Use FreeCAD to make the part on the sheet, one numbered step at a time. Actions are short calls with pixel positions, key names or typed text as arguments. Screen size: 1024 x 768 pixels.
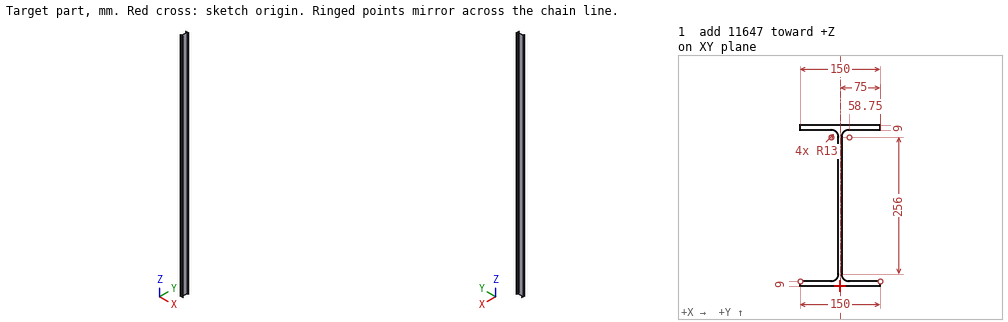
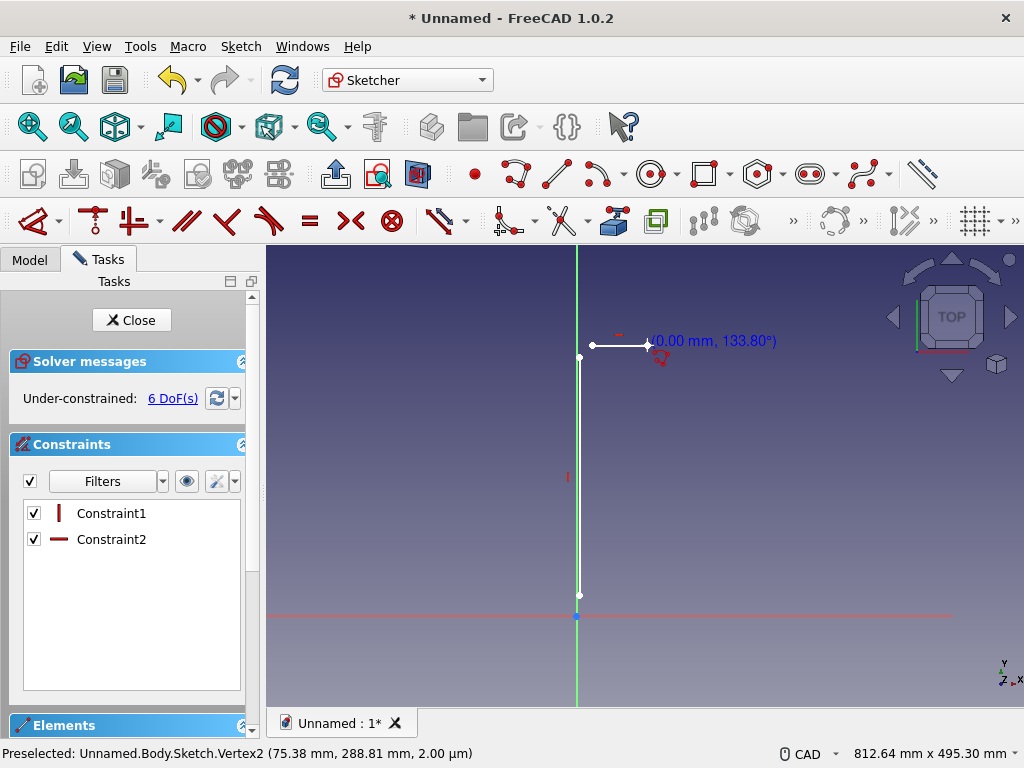
scroll(647, 337, up, 4)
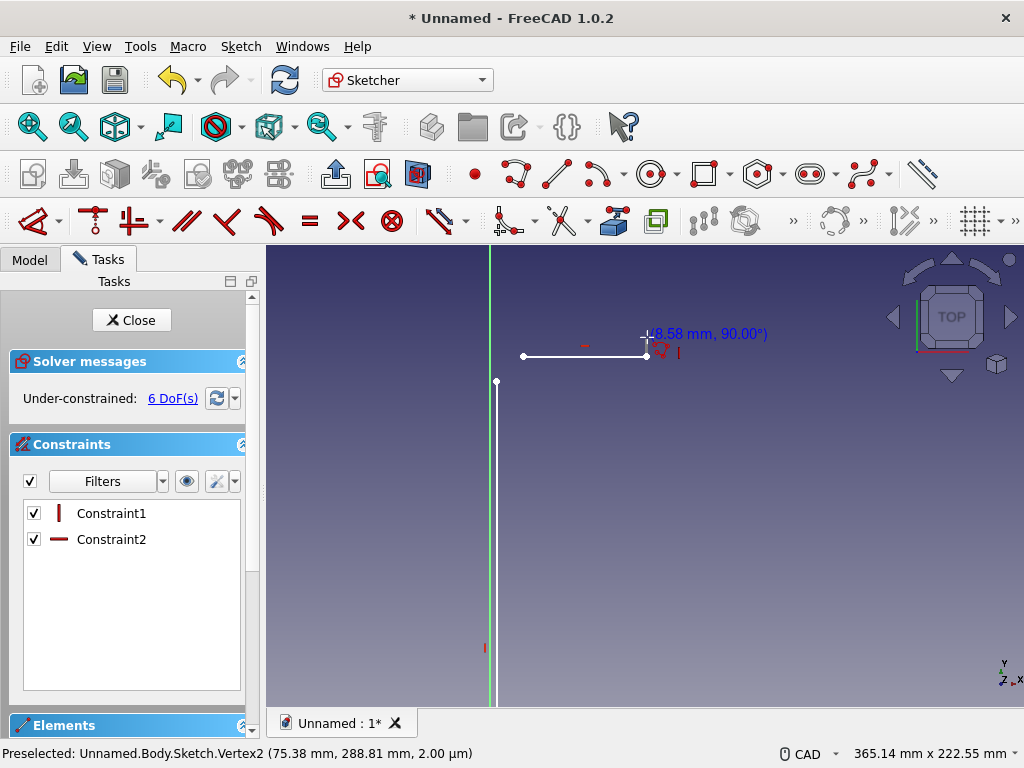
click(646, 336)
click(334, 336)
click(334, 354)
click(456, 354)
right_click(456, 354)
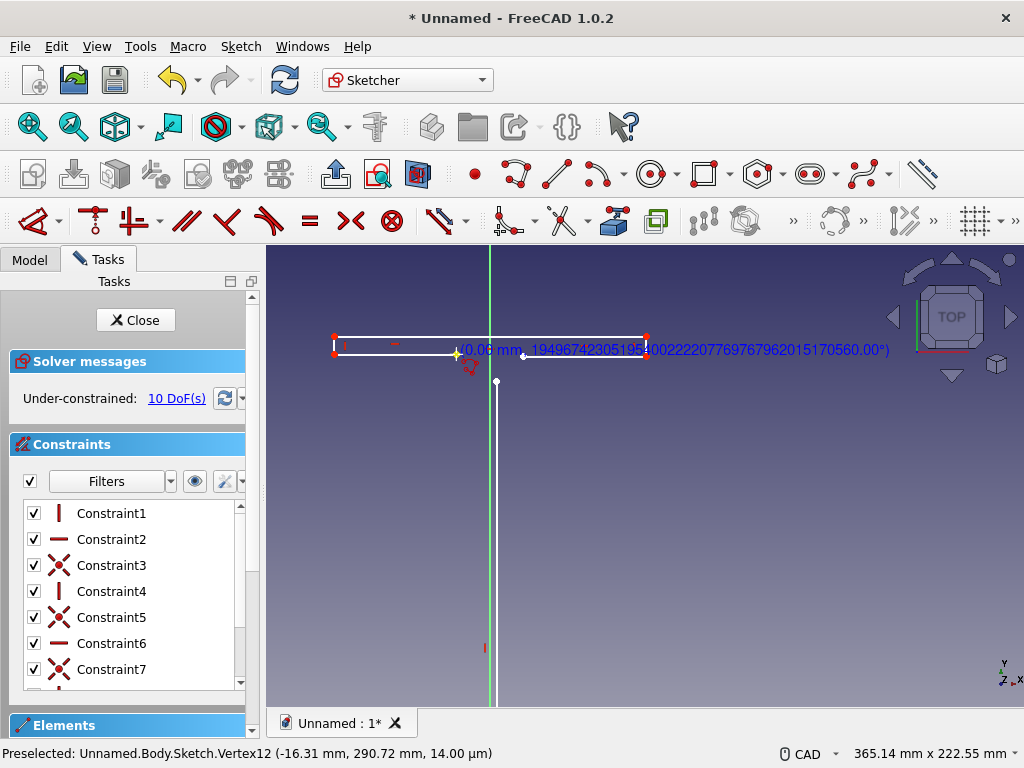
key(g)
key(l)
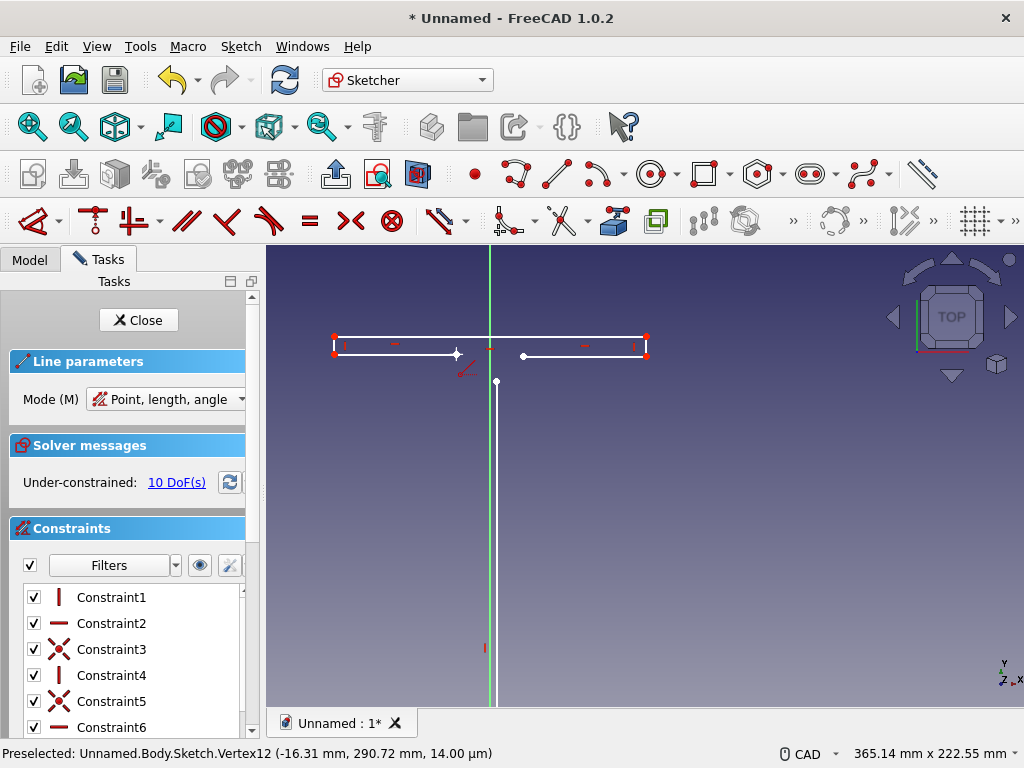
scroll(483, 381, up, 5)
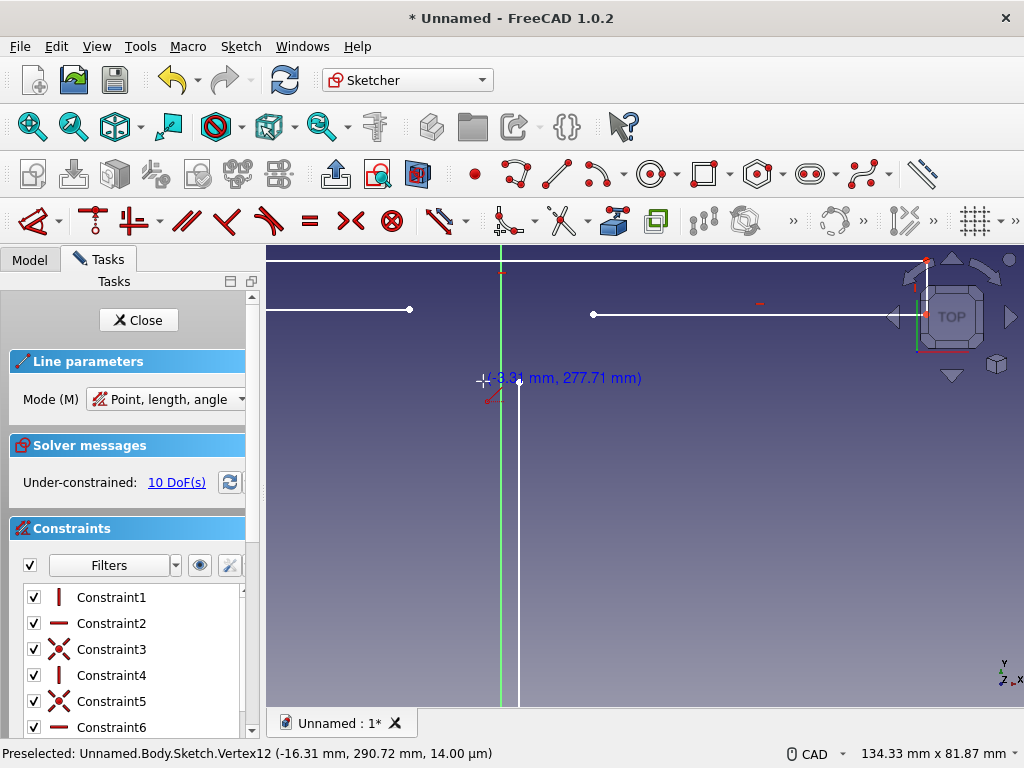
click(483, 382)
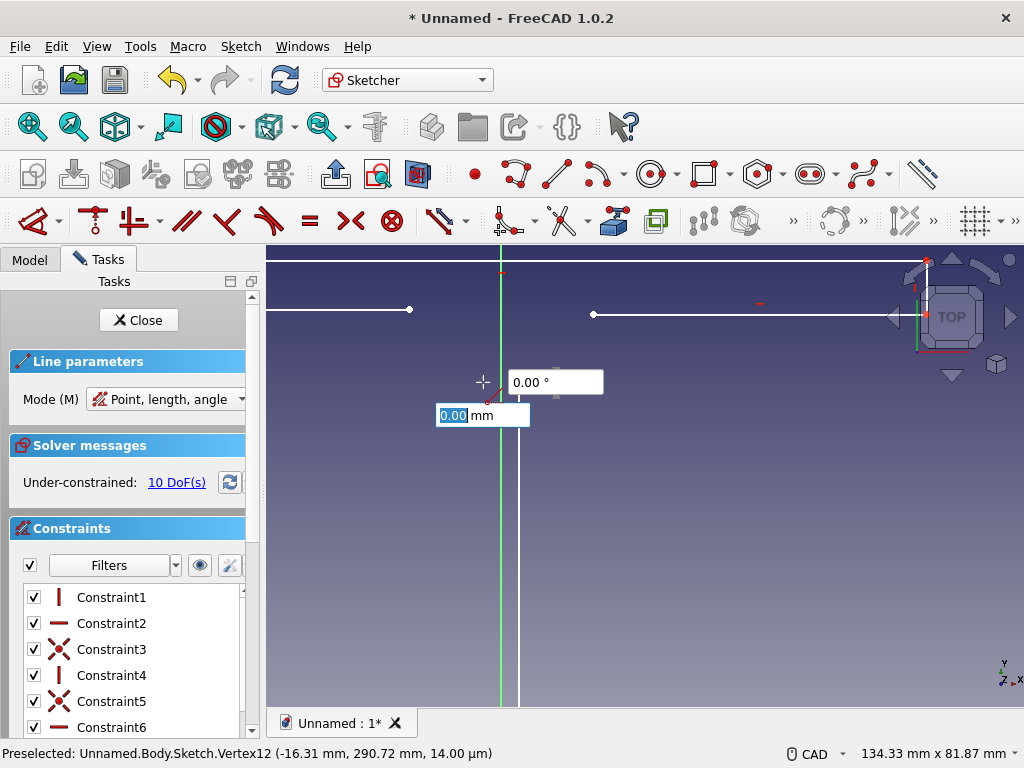
scroll(591, 352, down, 9)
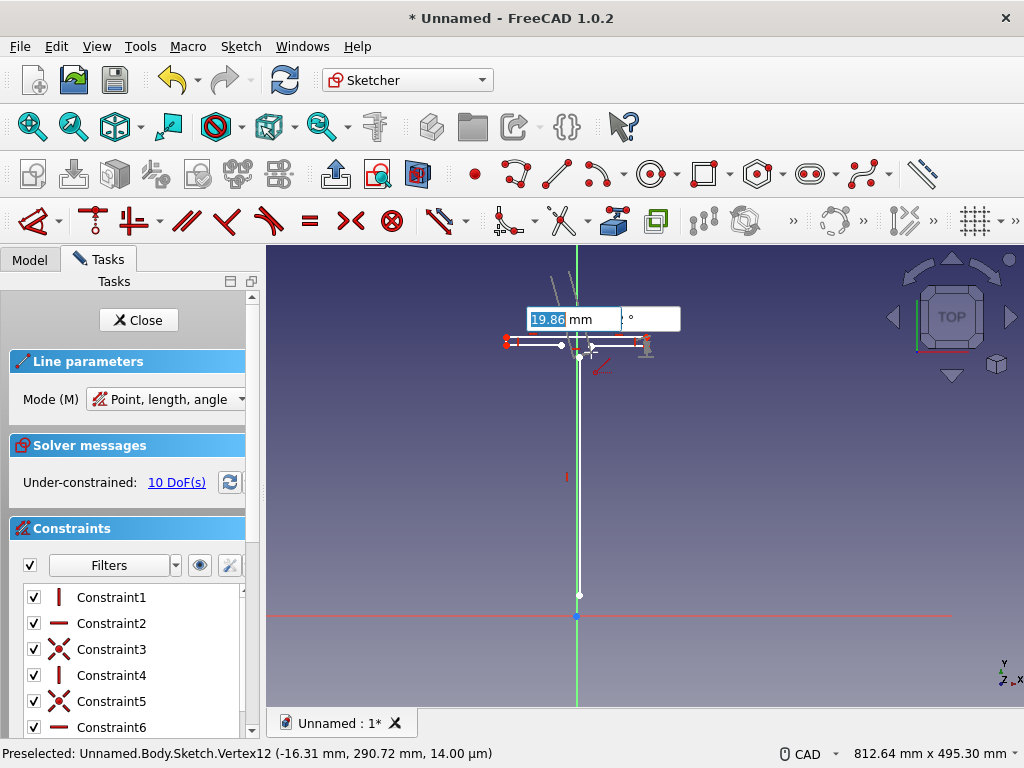
scroll(573, 596, up, 9)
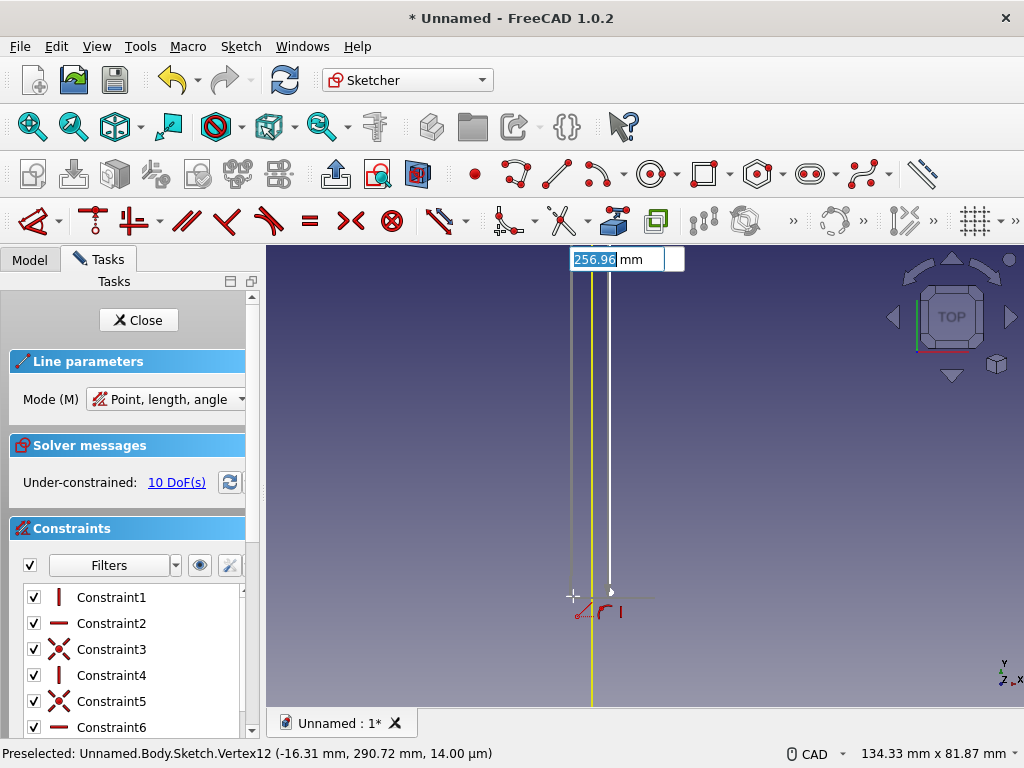
click(574, 591)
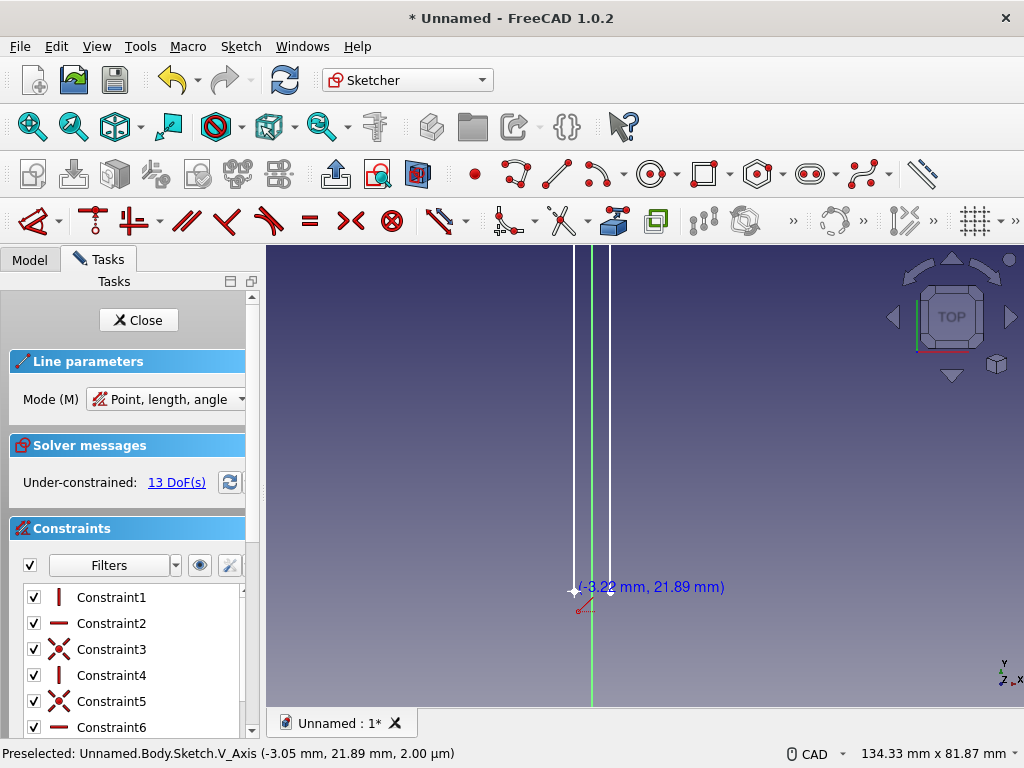
key(g)
key(m)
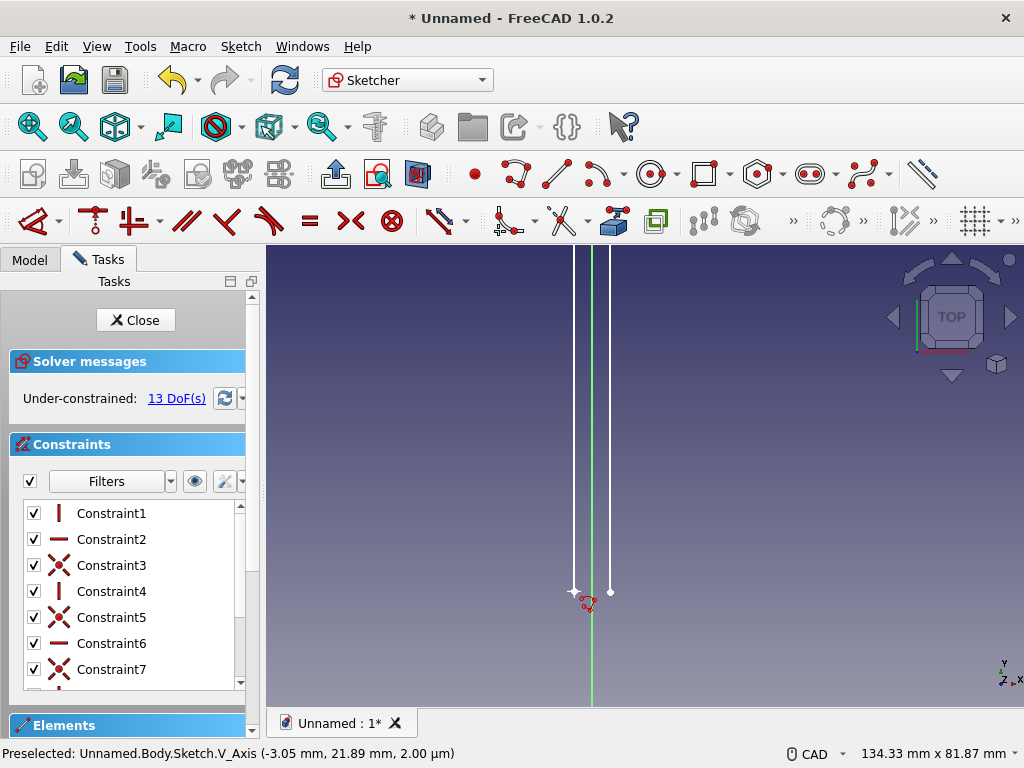
scroll(573, 596, down, 9)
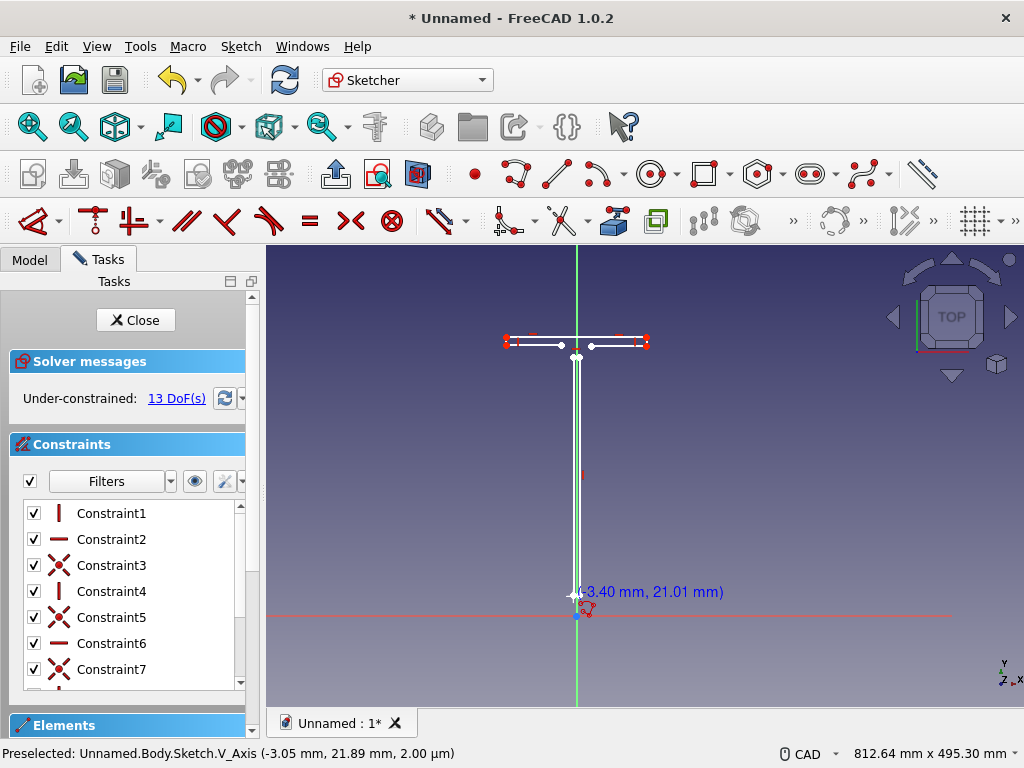
scroll(561, 608, up, 4)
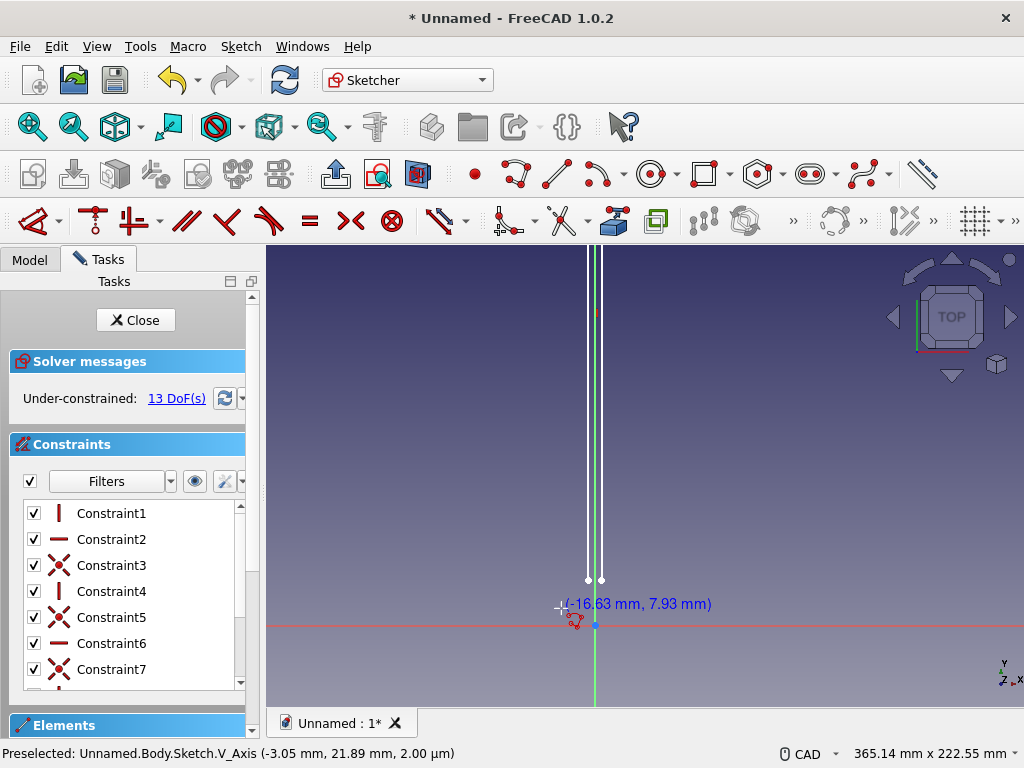
click(561, 607)
click(439, 607)
click(439, 626)
click(751, 617)
click(751, 607)
click(629, 607)
right_click(629, 607)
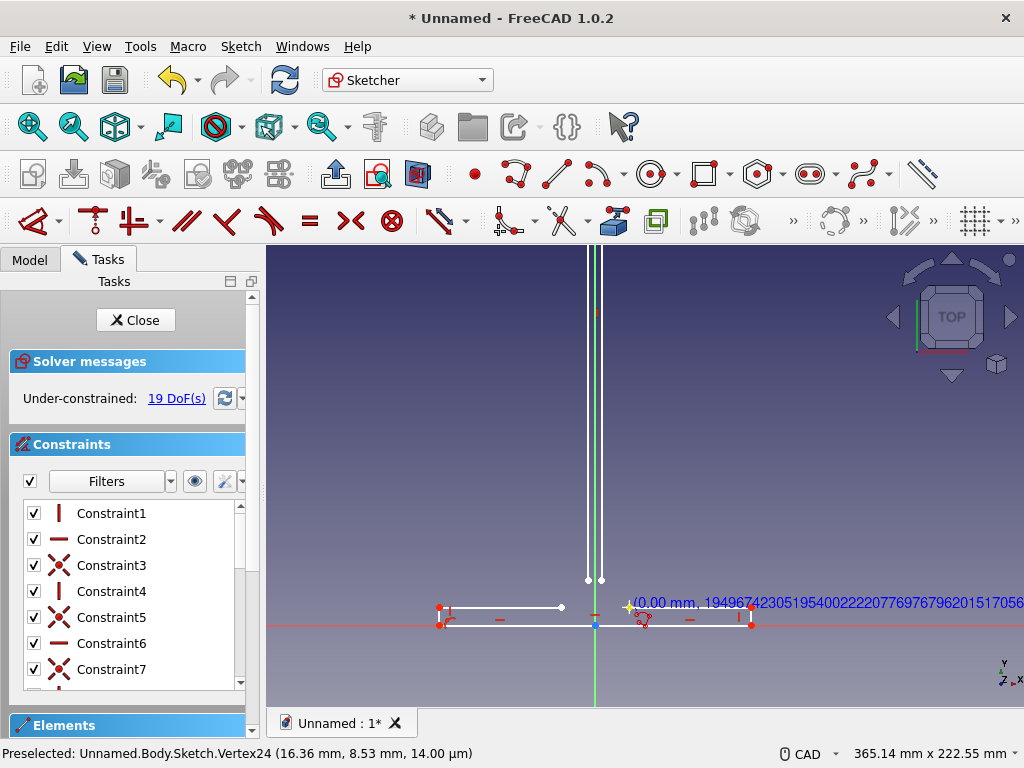
click(624, 174)